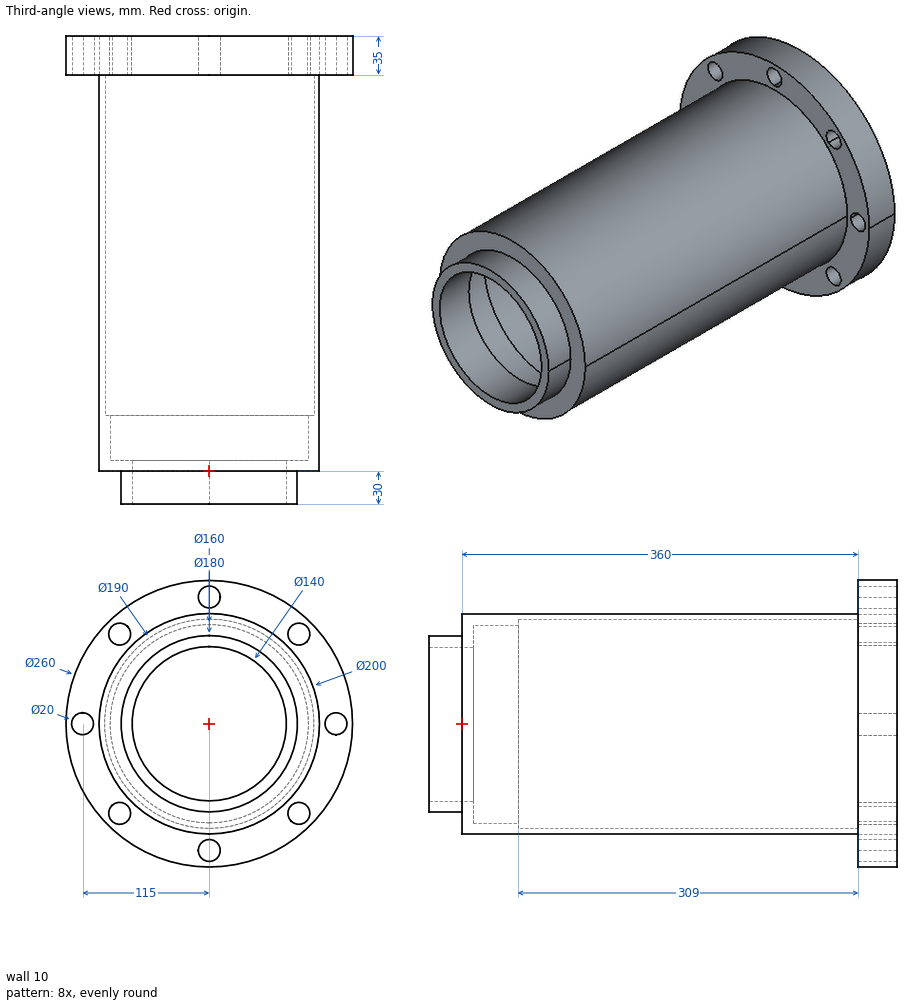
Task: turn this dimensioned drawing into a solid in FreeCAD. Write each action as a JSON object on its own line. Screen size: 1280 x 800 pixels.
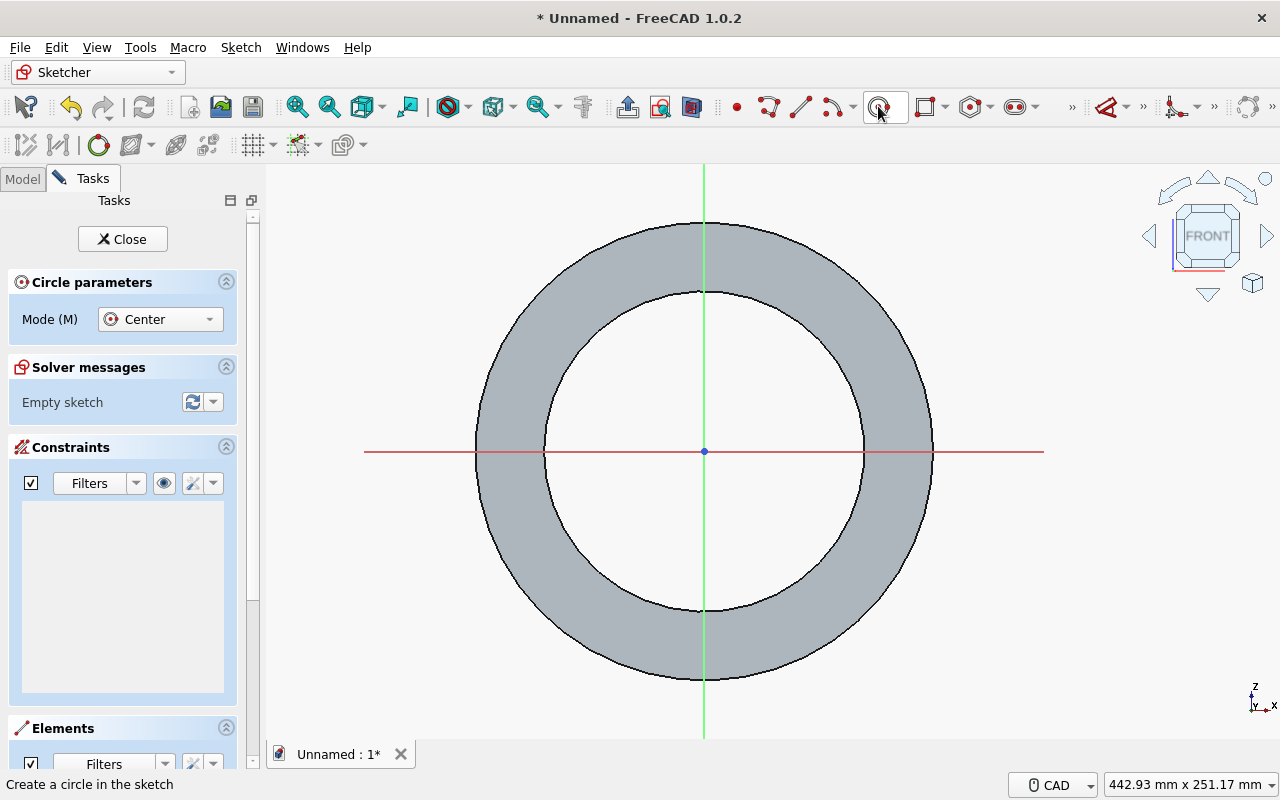
{"action": "left_click", "coordinate": [704, 452]}
{"action": "left_click", "coordinate": [834, 322]}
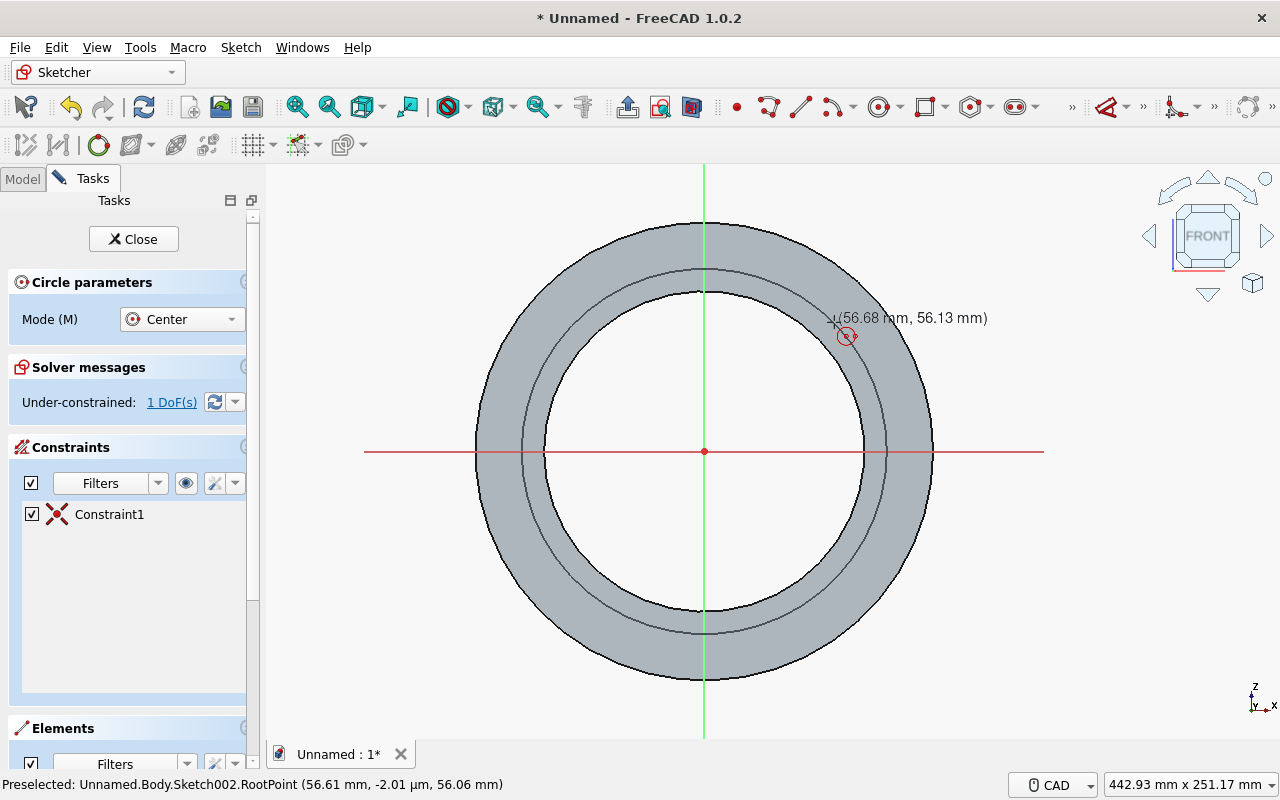
{"action": "left_click", "coordinate": [704, 452]}
{"action": "left_click", "coordinate": [818, 338]}
{"action": "key", "text": "Escape"}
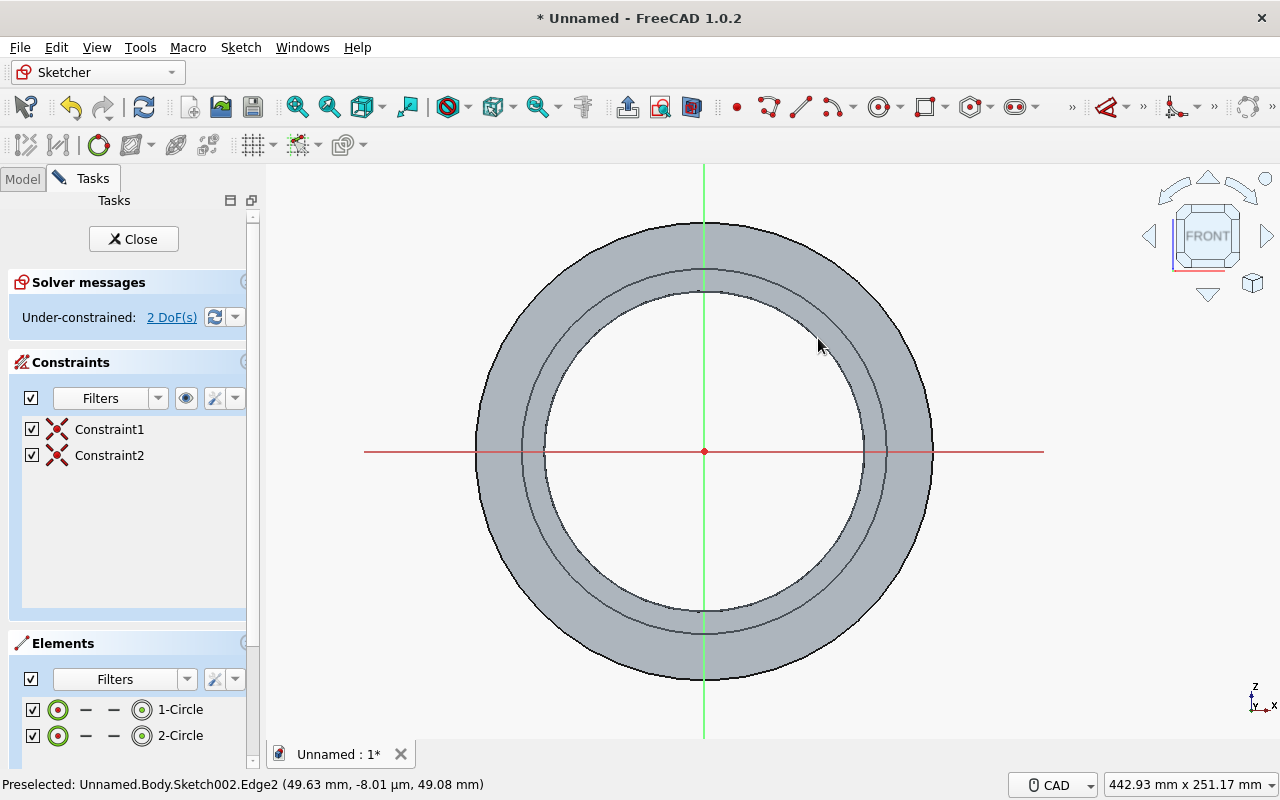
{"action": "key", "text": "d"}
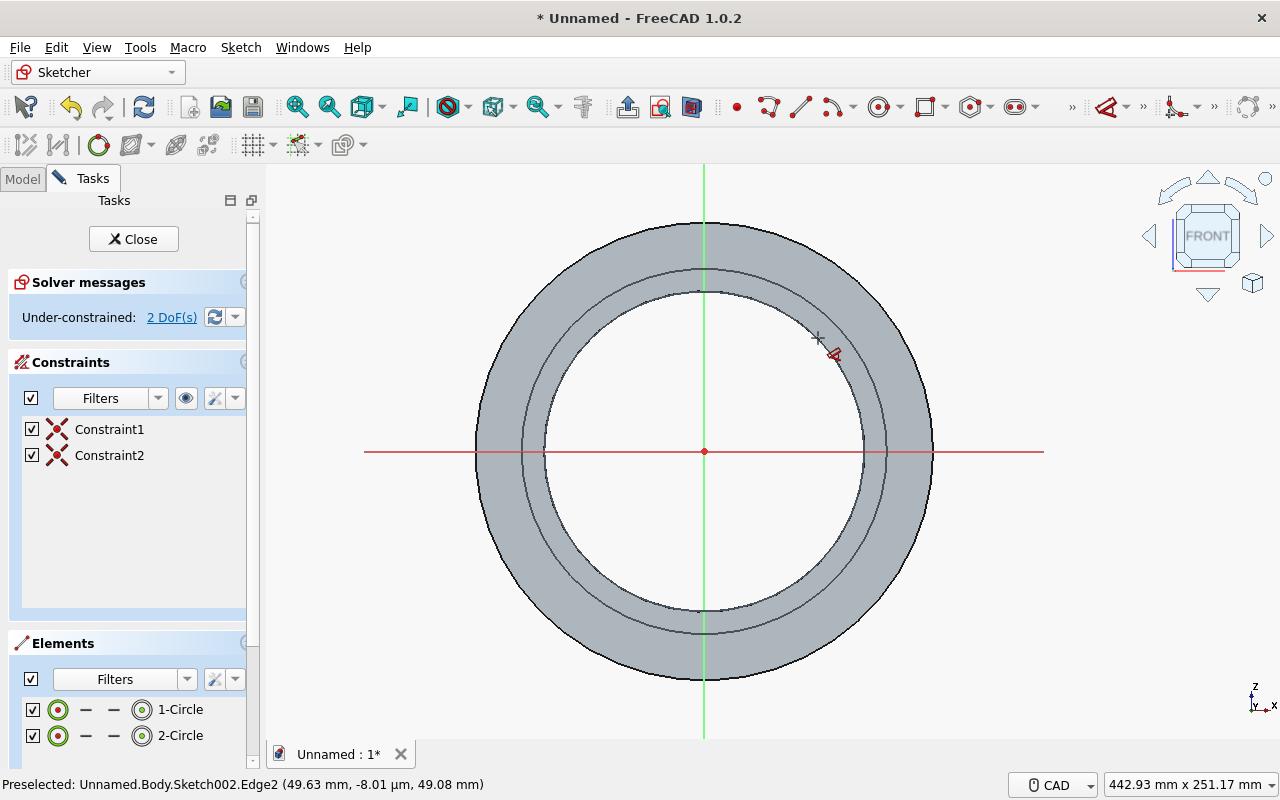
{"action": "left_click", "coordinate": [833, 322]}
{"action": "left_click", "coordinate": [856, 299]}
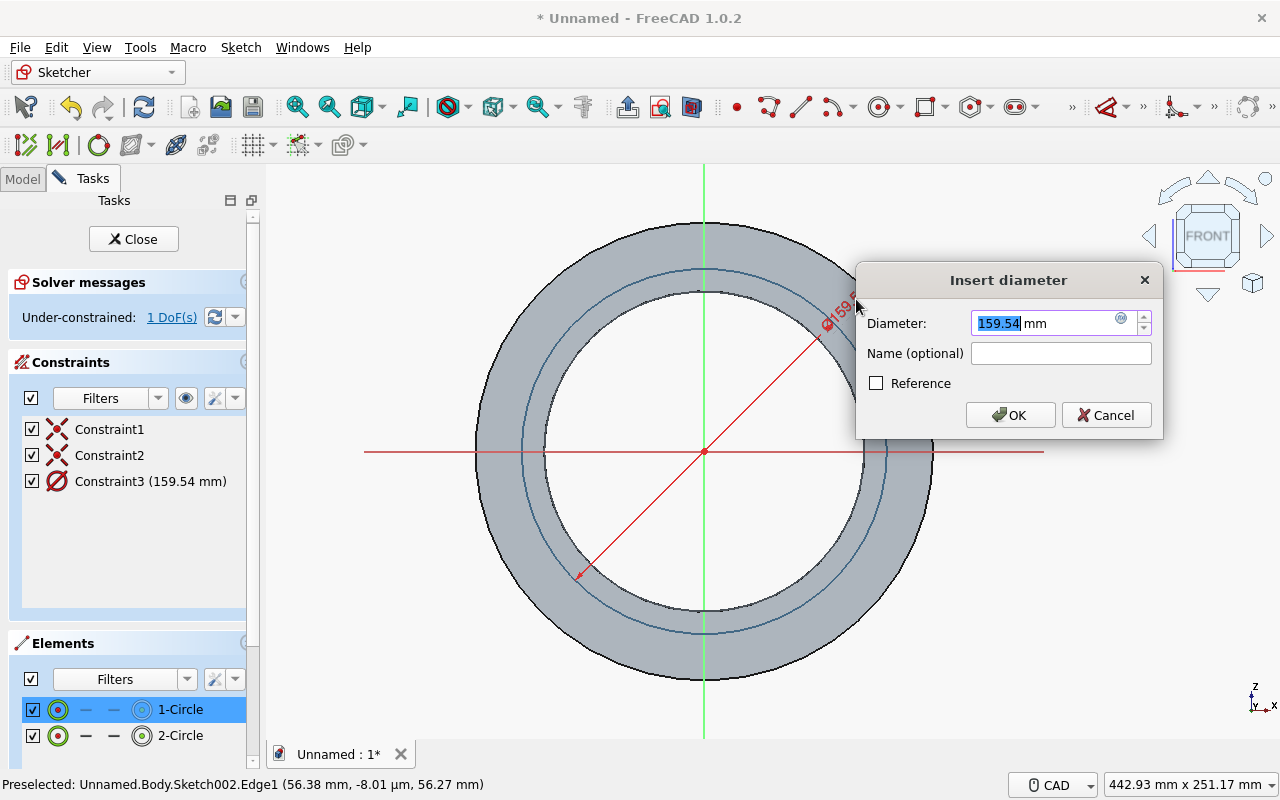
{"action": "type", "text": "160"}
{"action": "key", "text": "Return"}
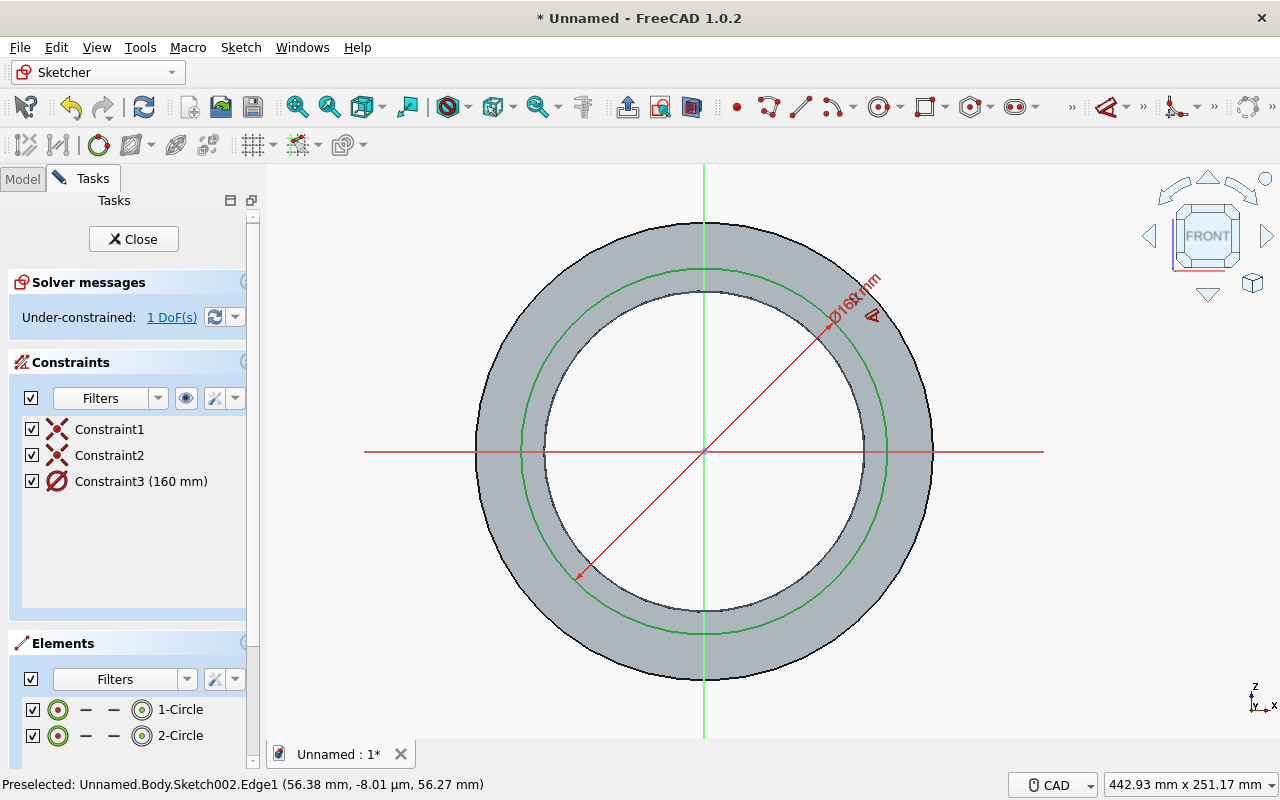
{"action": "left_click", "coordinate": [817, 338]}
{"action": "left_click", "coordinate": [910, 390]}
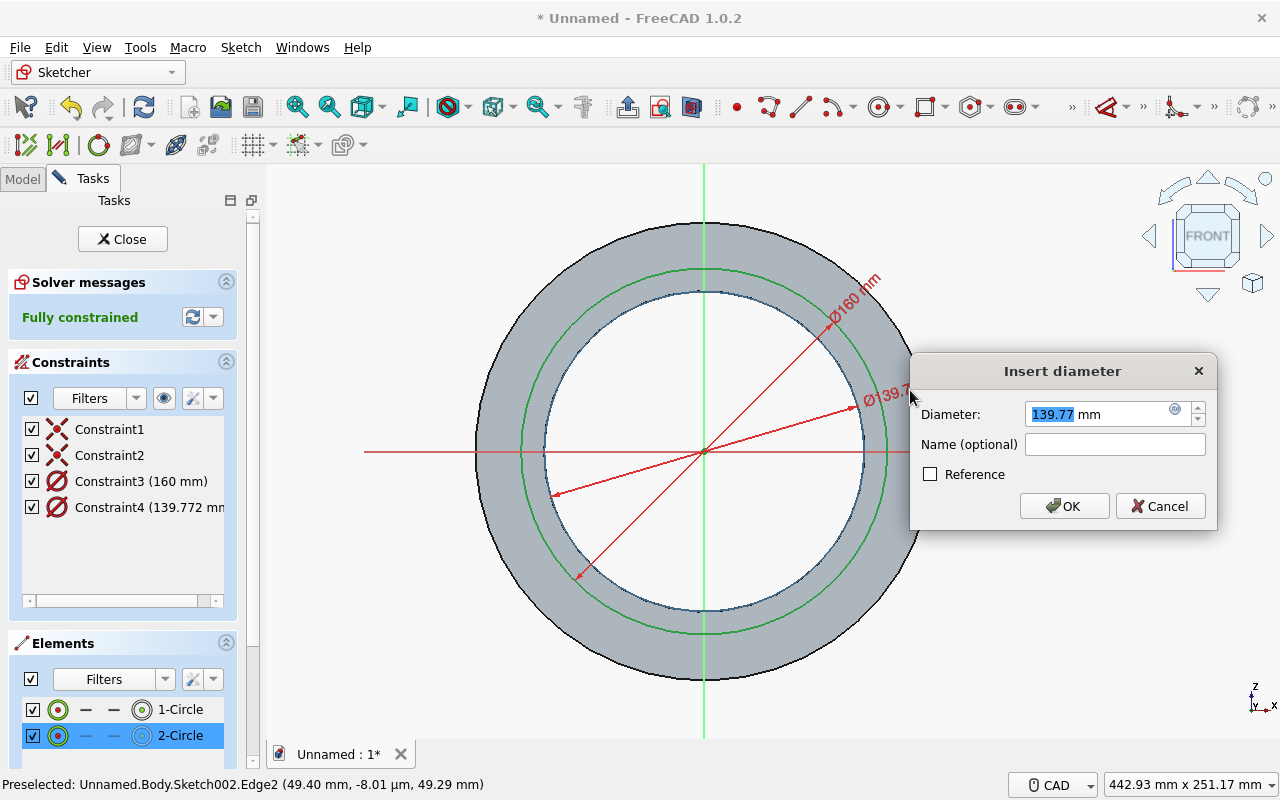
{"action": "type", "text": "140"}
{"action": "key", "text": "Return"}
{"action": "key", "text": "Escape"}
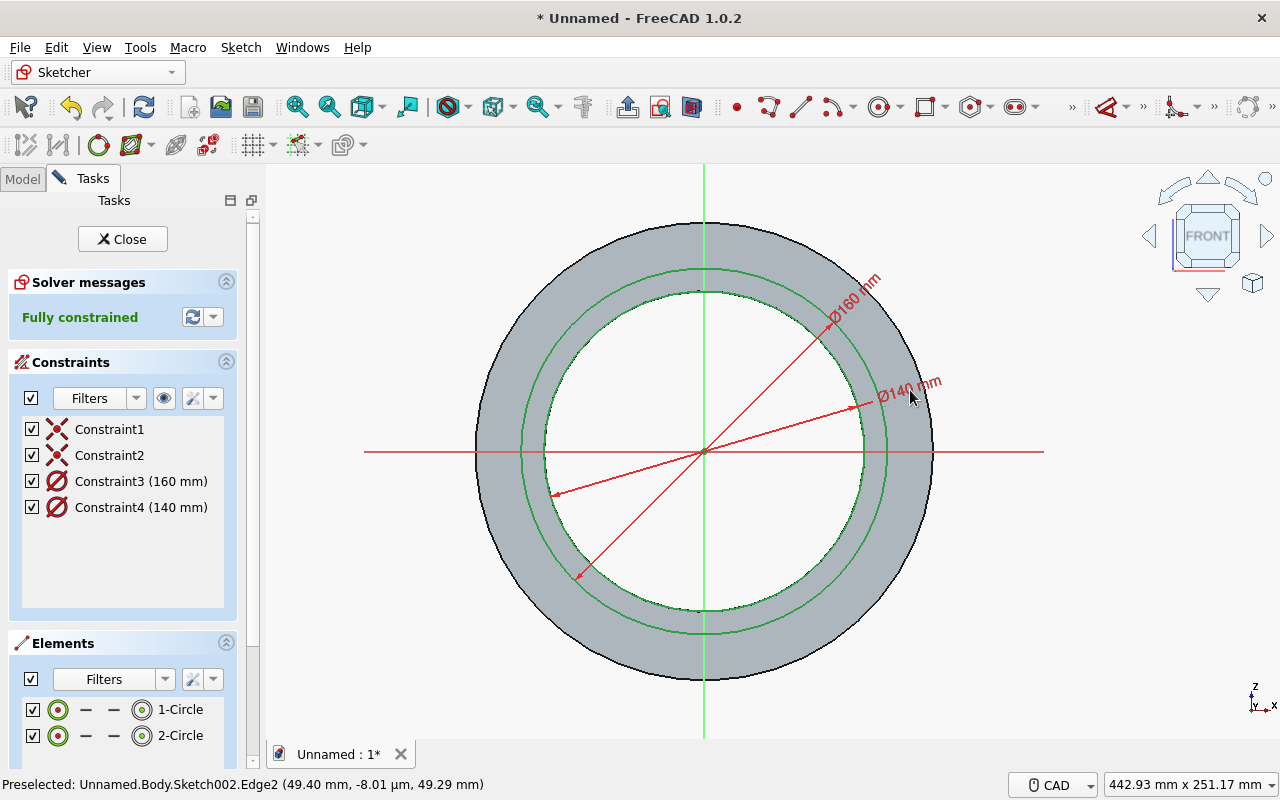
{"action": "left_click", "coordinate": [123, 239]}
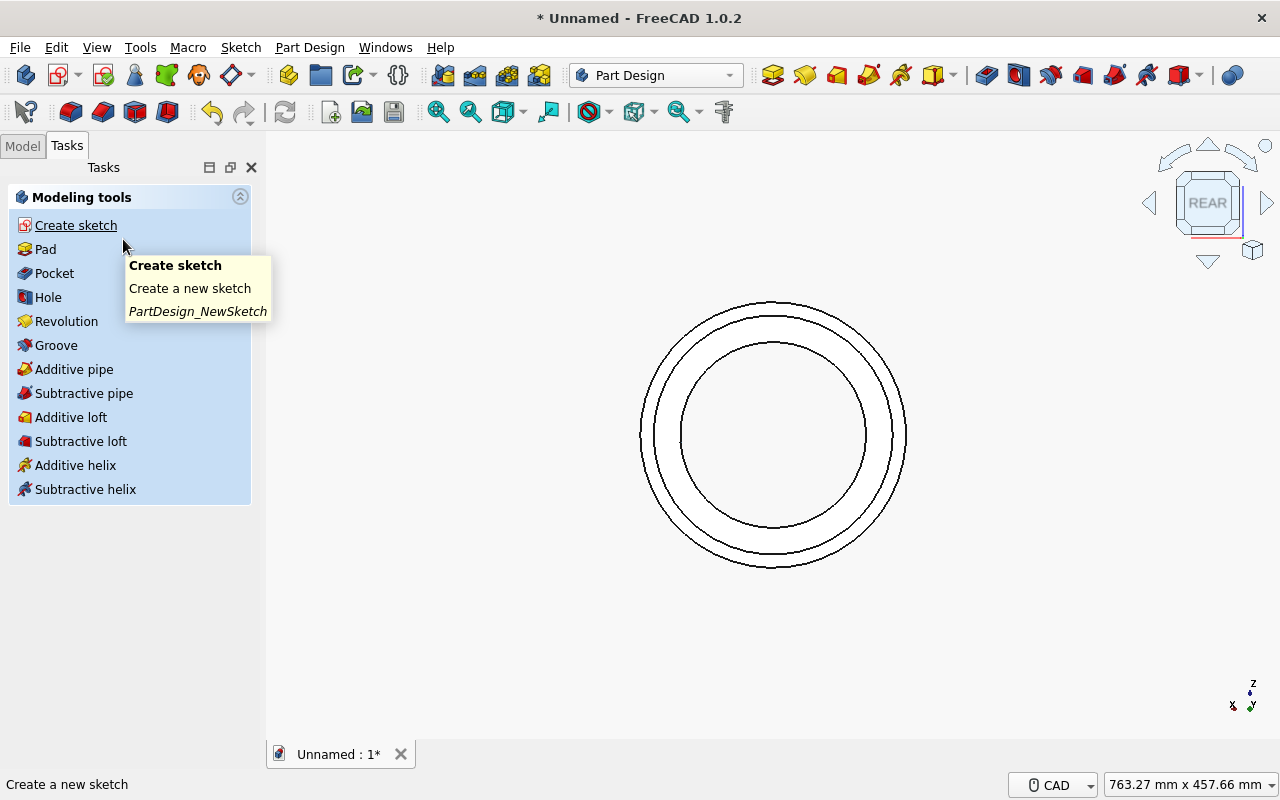
{"action": "left_click", "coordinate": [774, 76]}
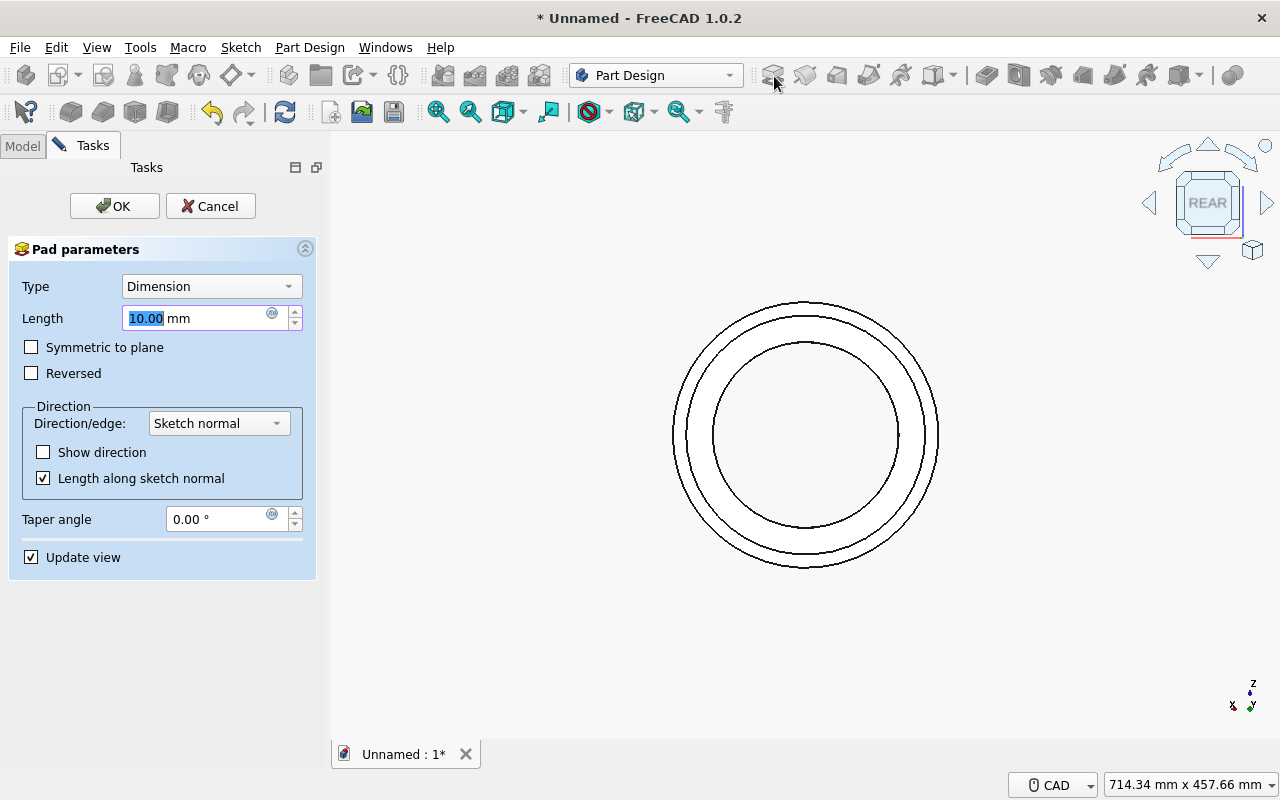
{"action": "type", "text": "30"}
{"action": "key", "text": "Tab"}